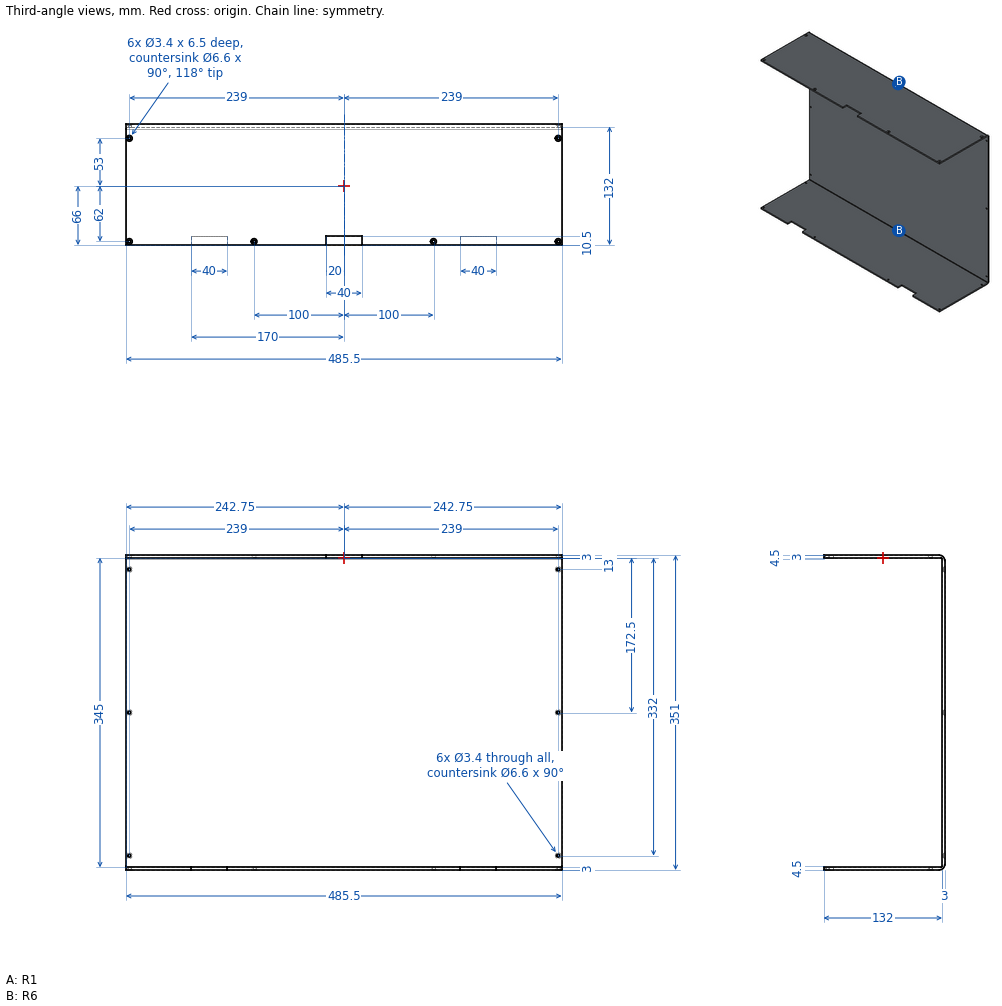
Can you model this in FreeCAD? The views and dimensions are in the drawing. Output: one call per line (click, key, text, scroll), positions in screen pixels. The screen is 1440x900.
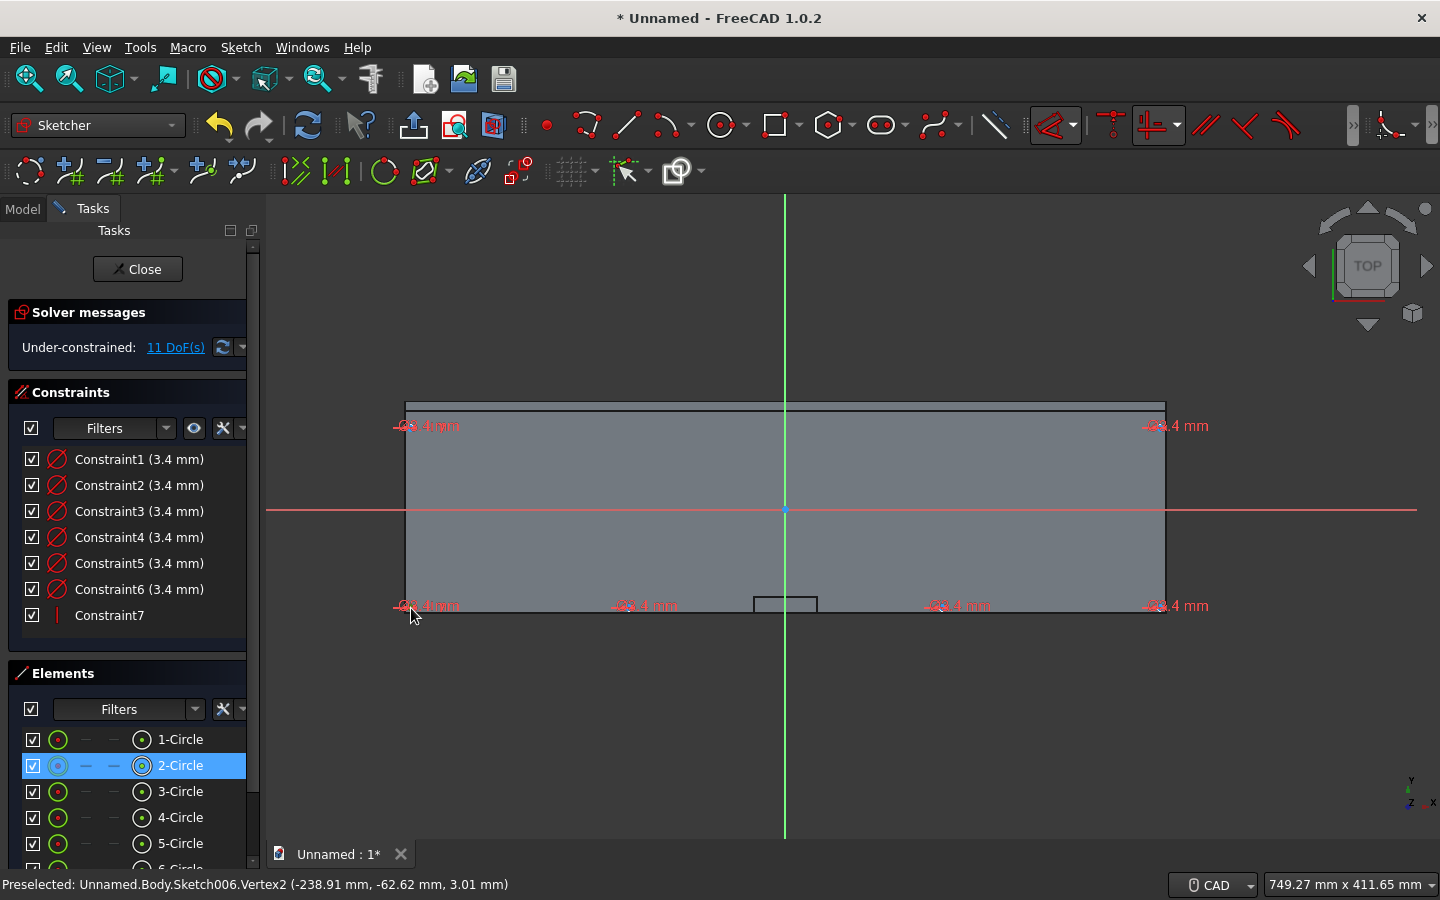
click(629, 608)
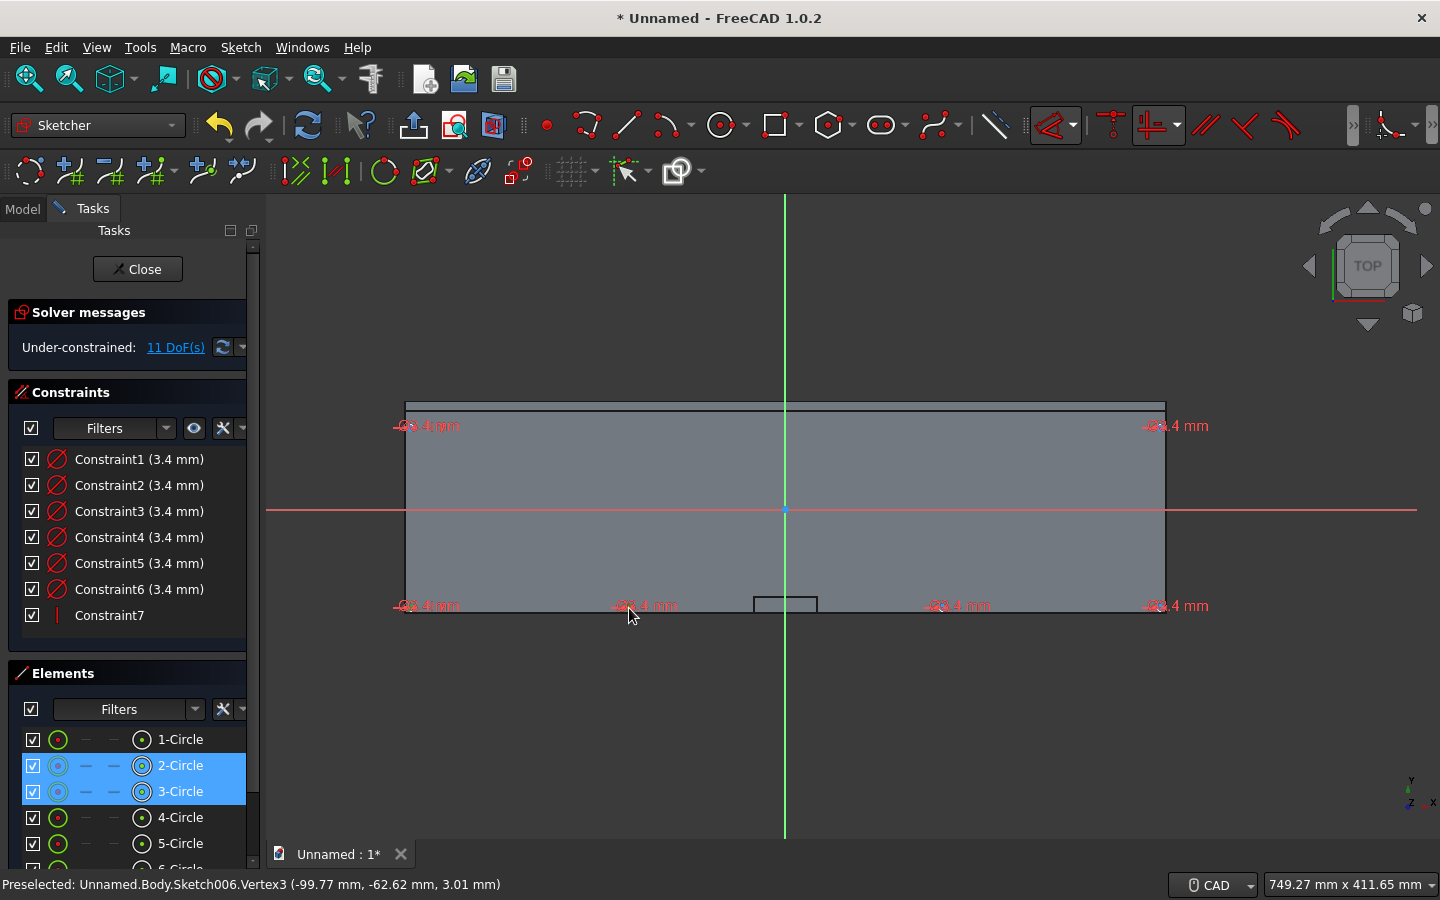
click(1180, 126)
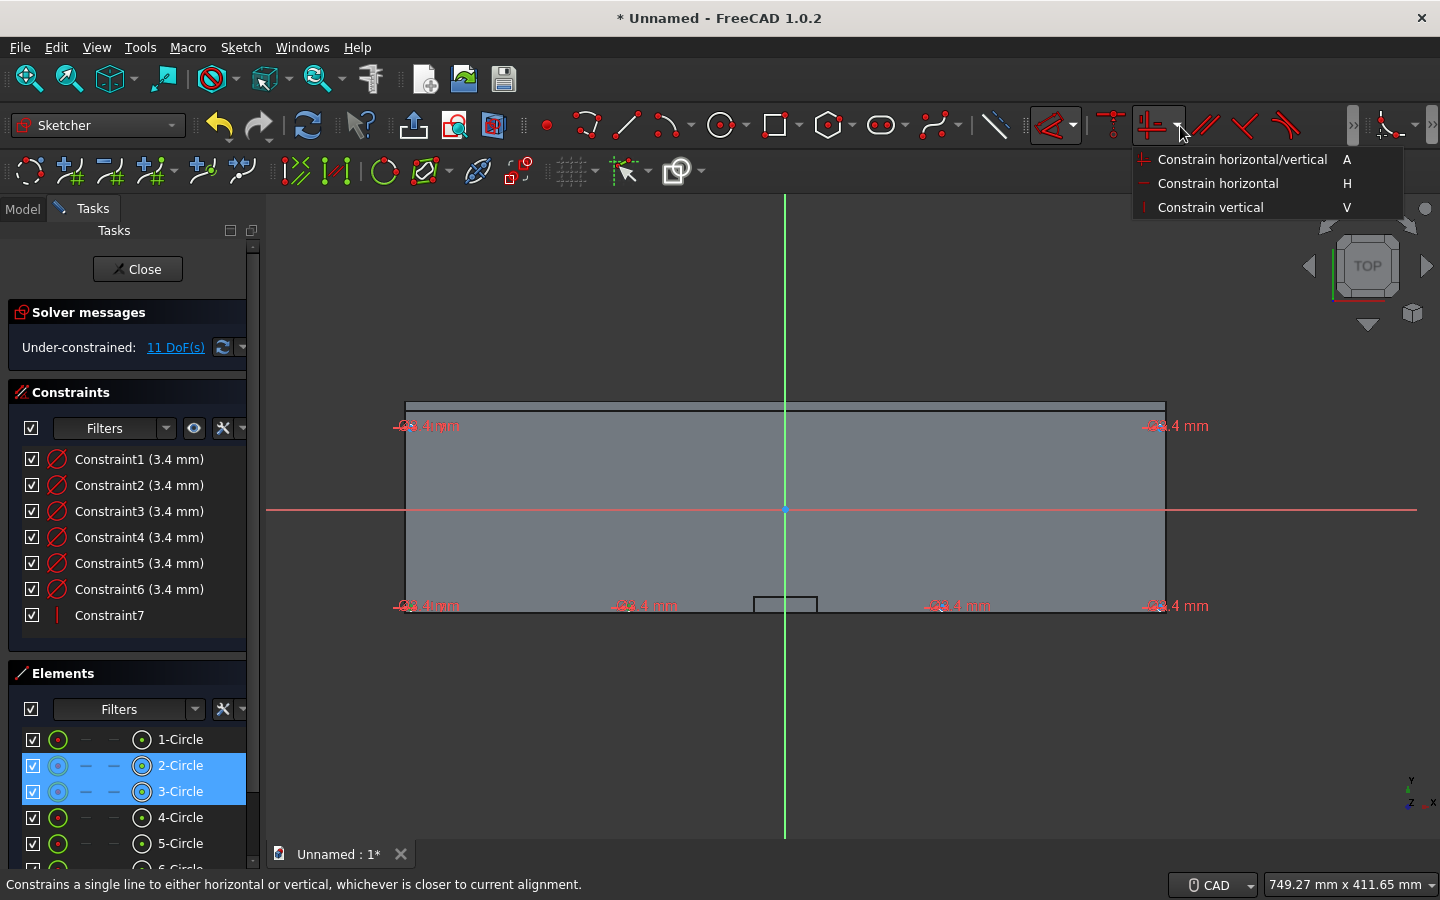
click(1268, 183)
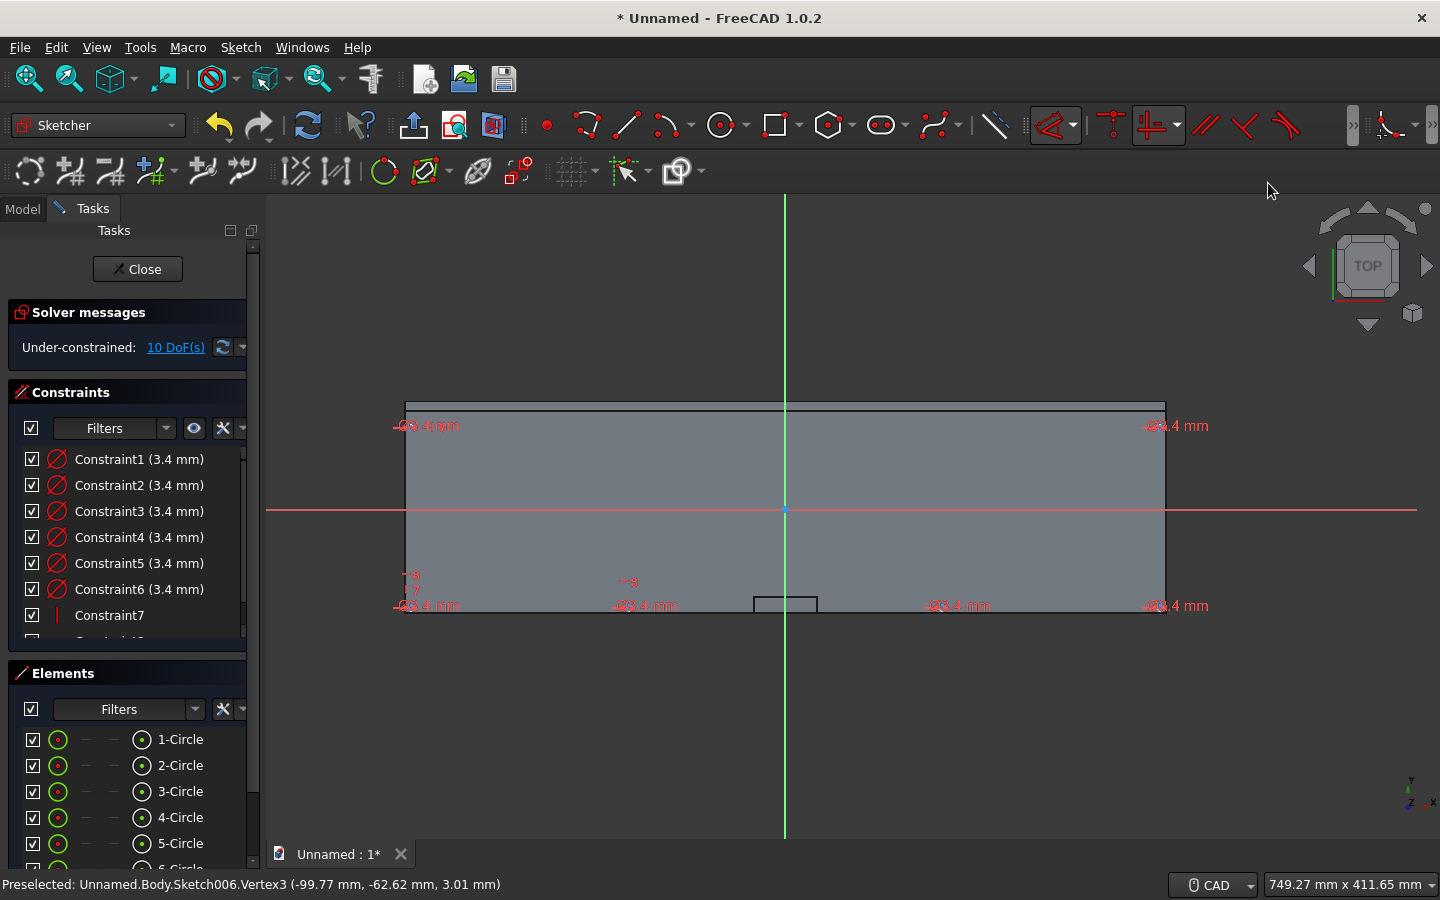
click(629, 608)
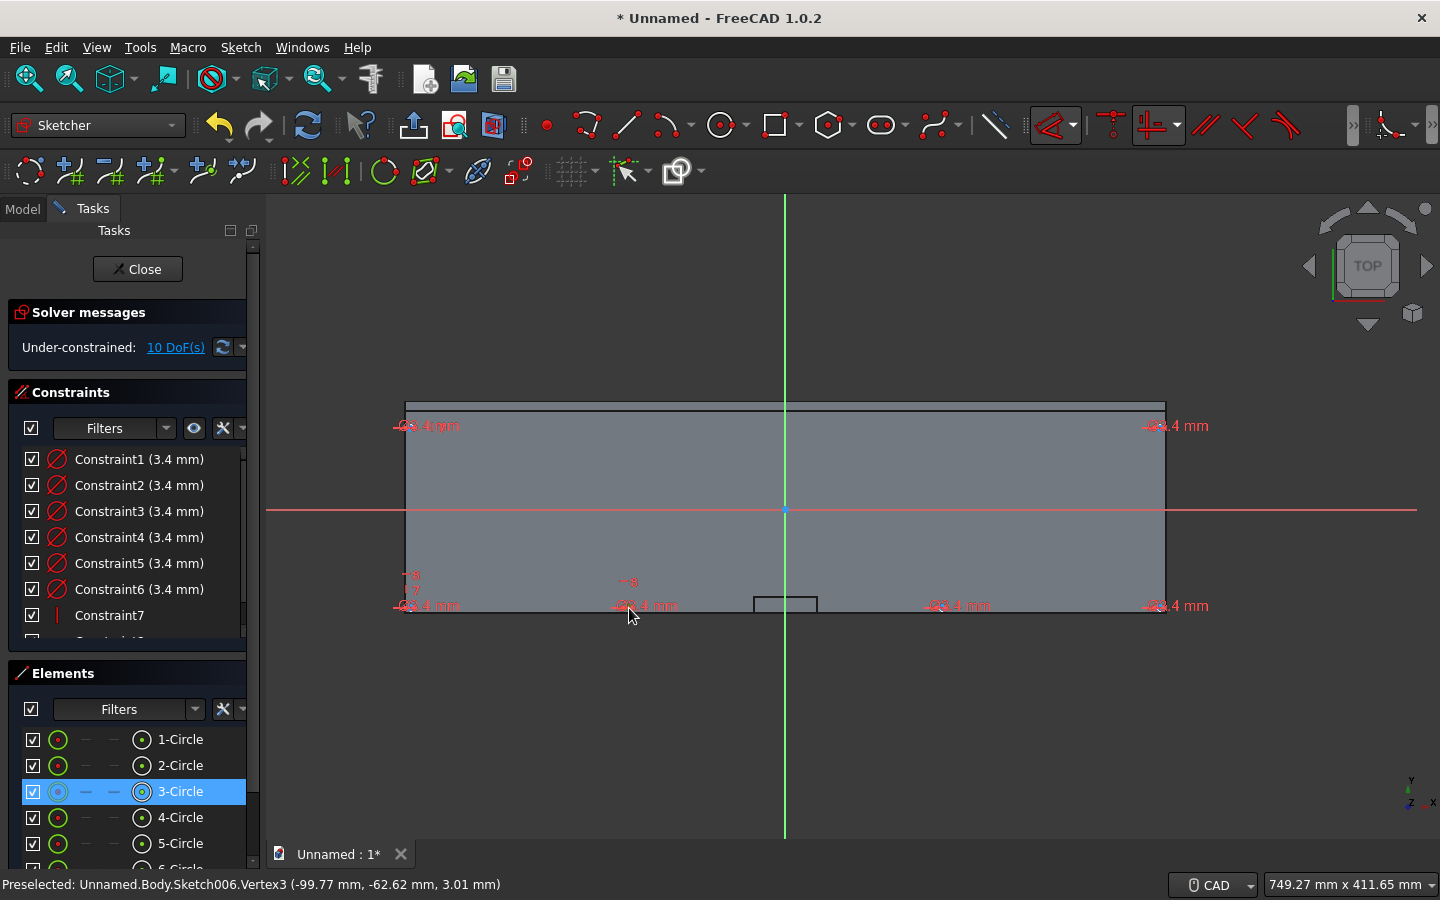
click(942, 608)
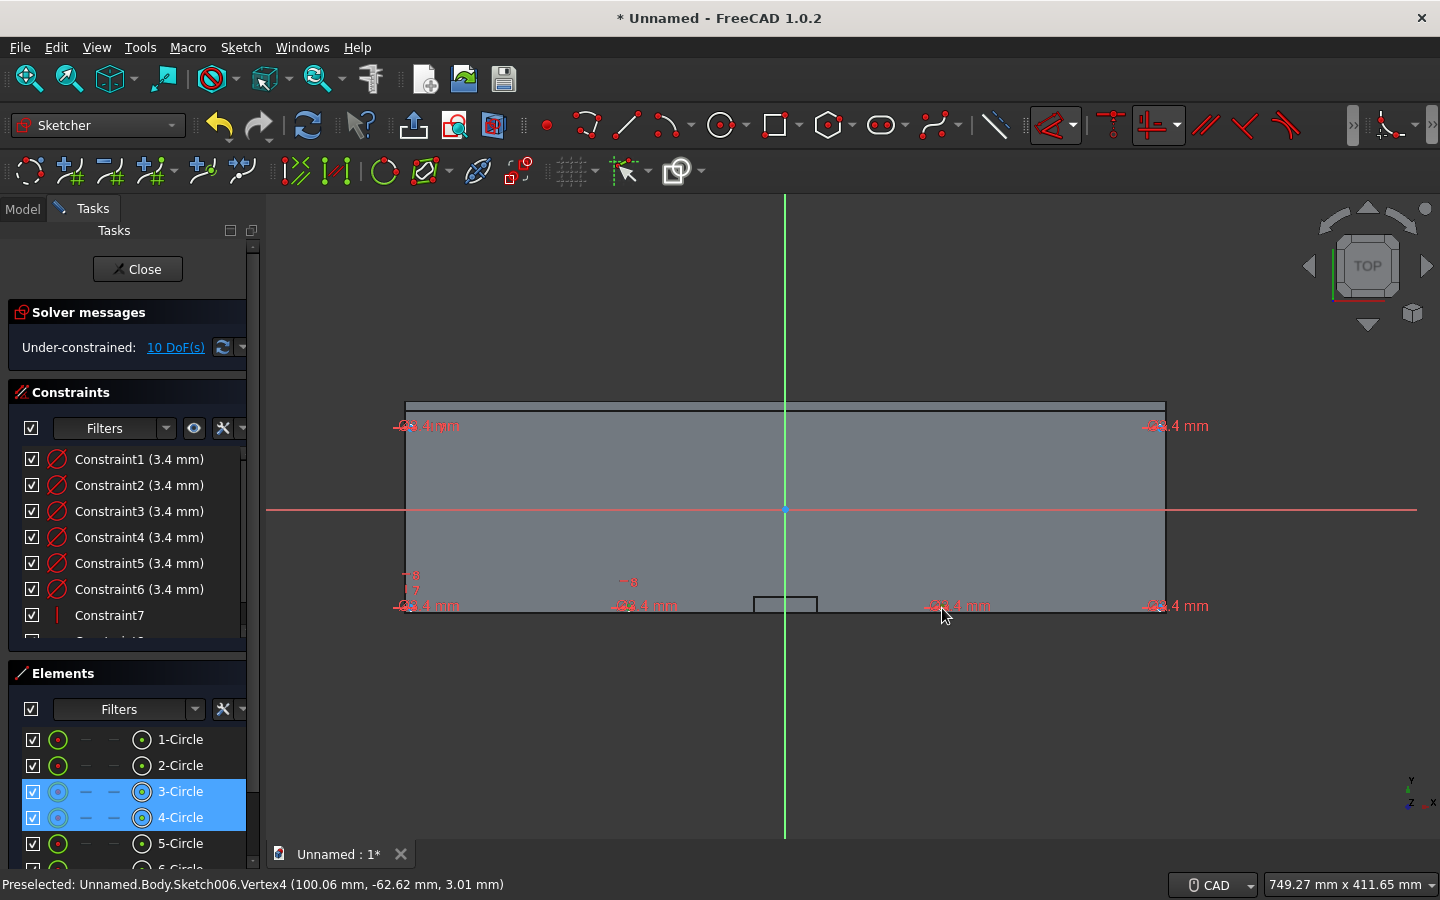
key(h)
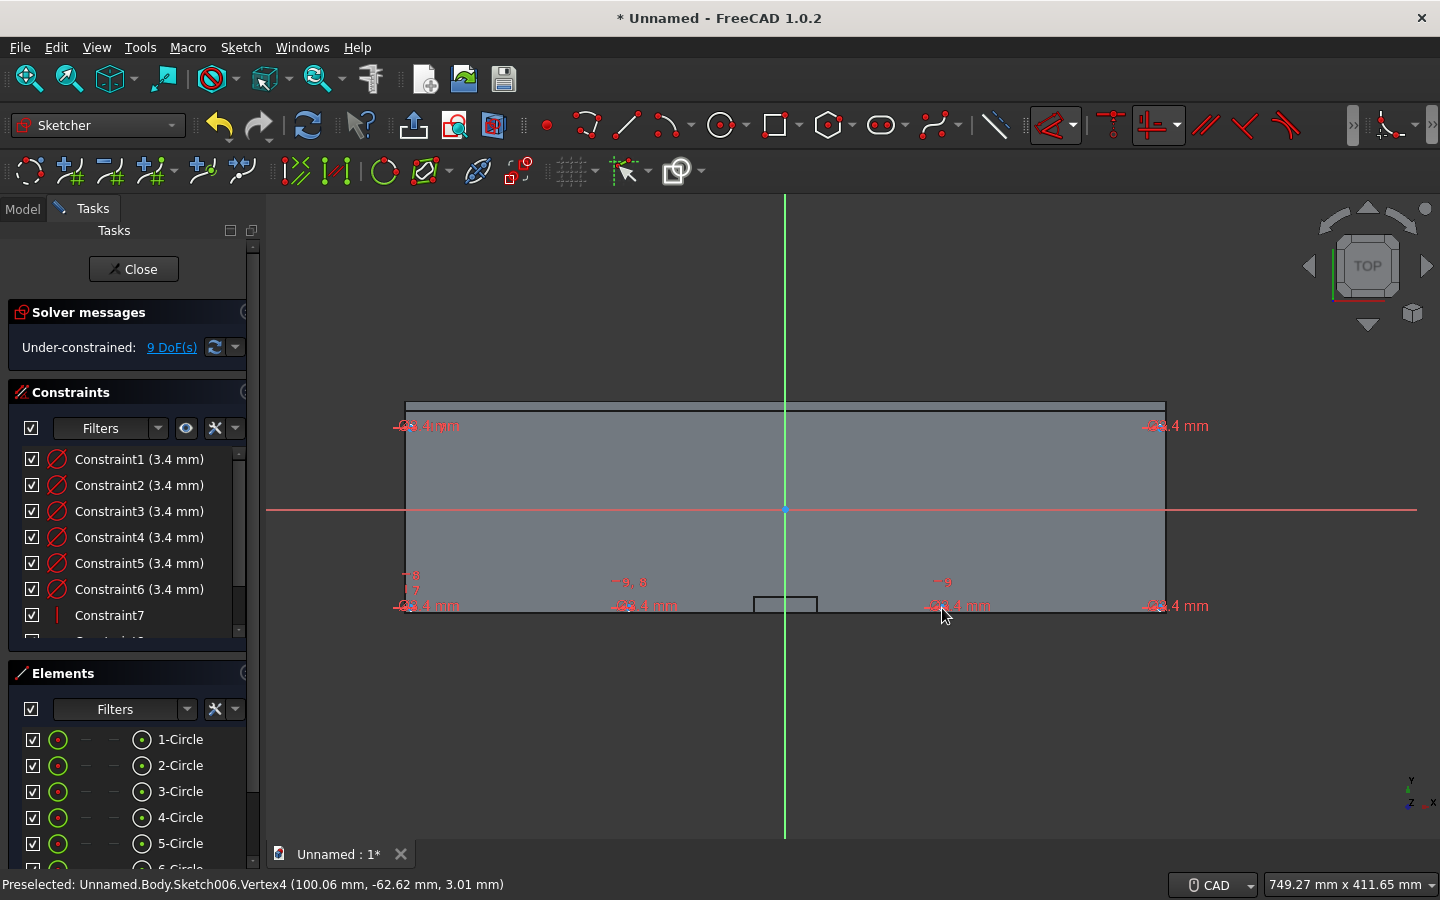
click(411, 428)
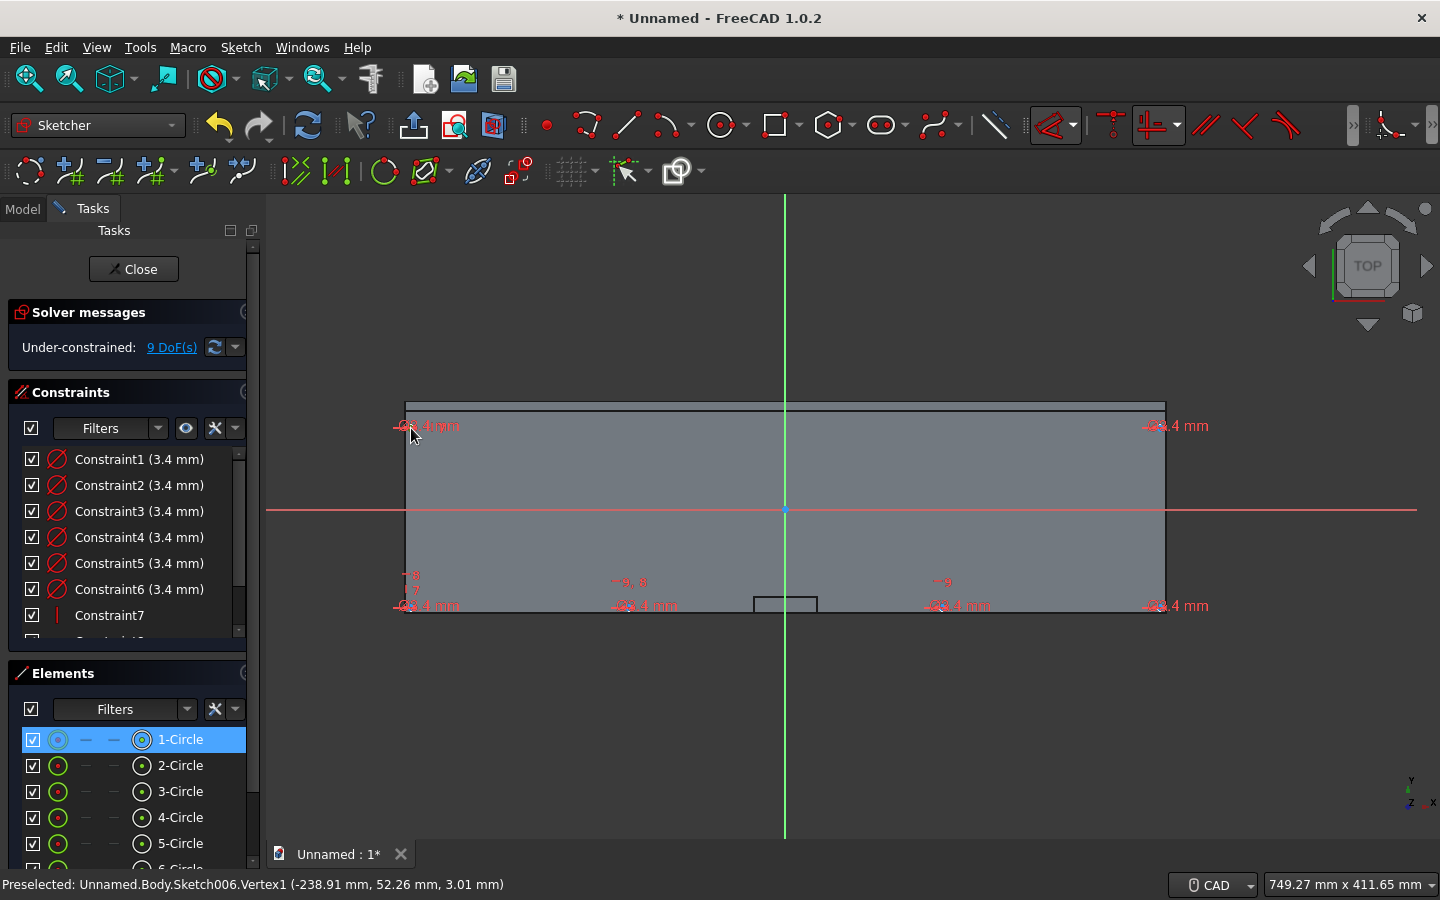
click(1160, 428)